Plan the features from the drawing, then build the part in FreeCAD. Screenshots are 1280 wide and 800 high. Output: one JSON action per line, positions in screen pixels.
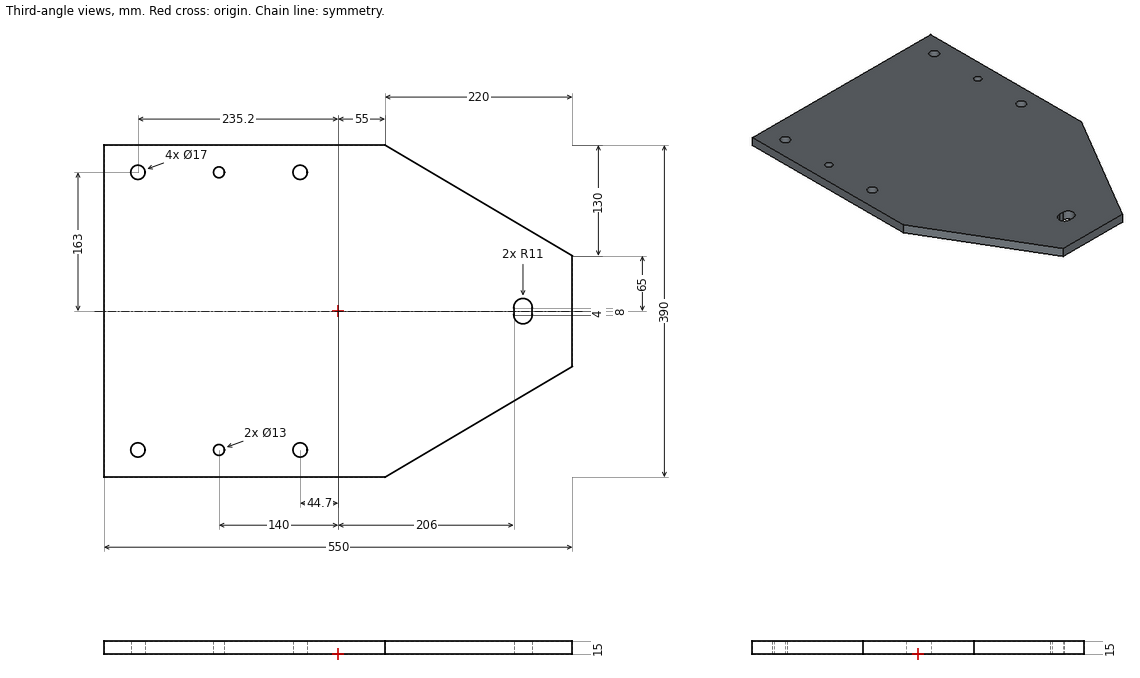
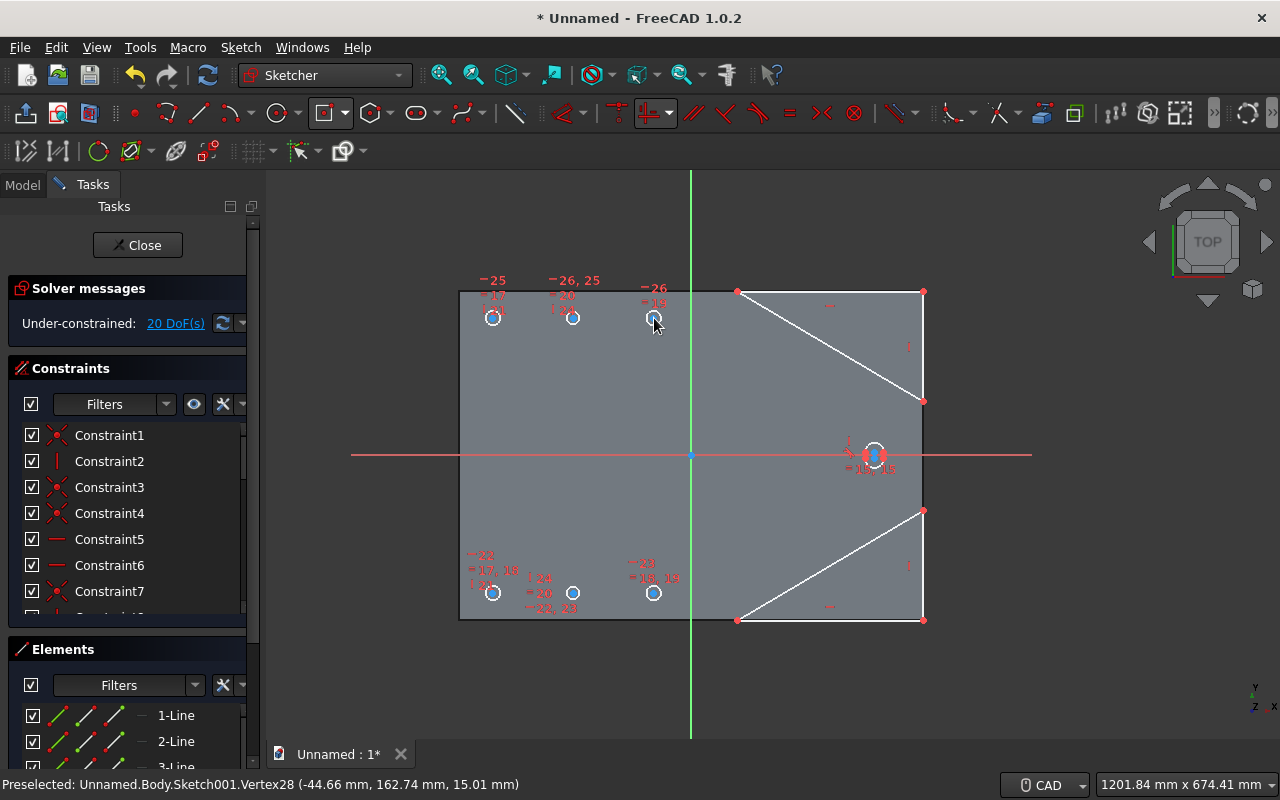
{"action": "left_click", "coordinate": [654, 593]}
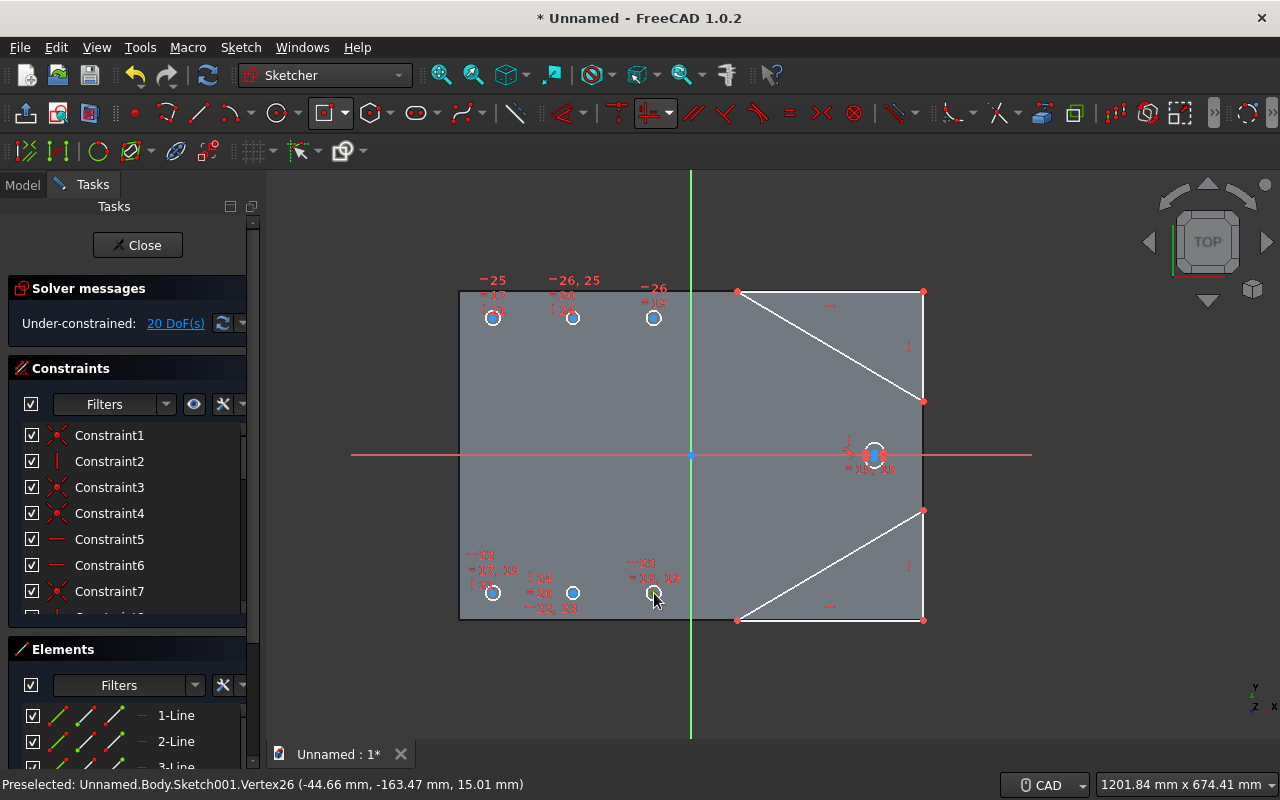
{"action": "left_click", "coordinate": [654, 318]}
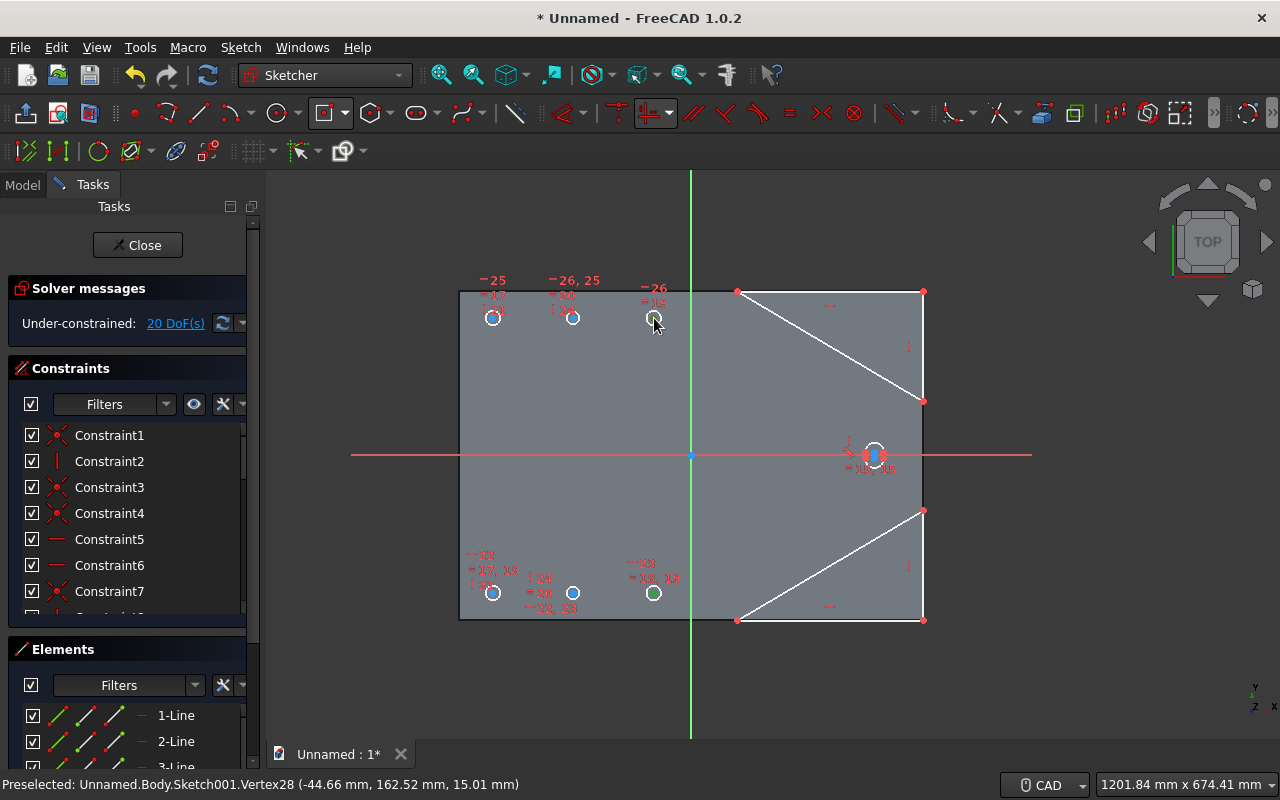
{"action": "left_click", "coordinate": [353, 455]}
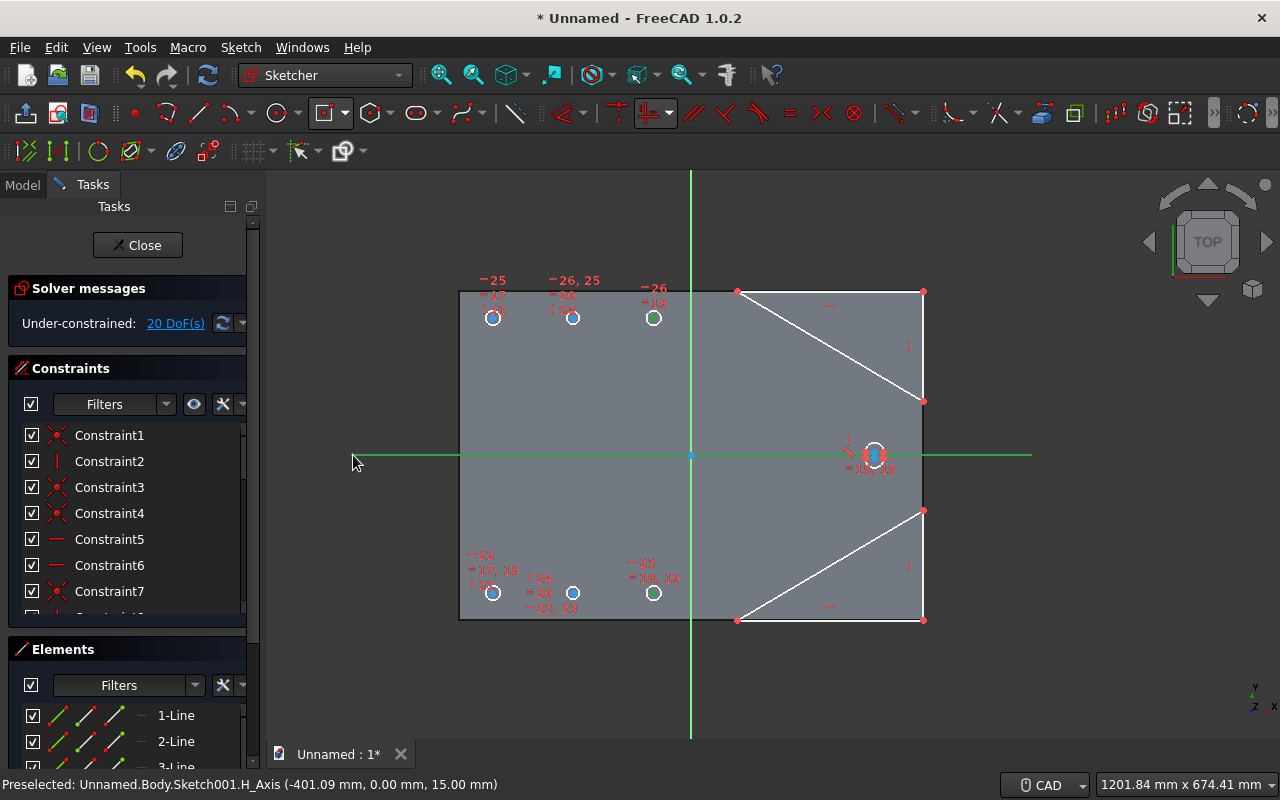
{"action": "left_click", "coordinate": [822, 114]}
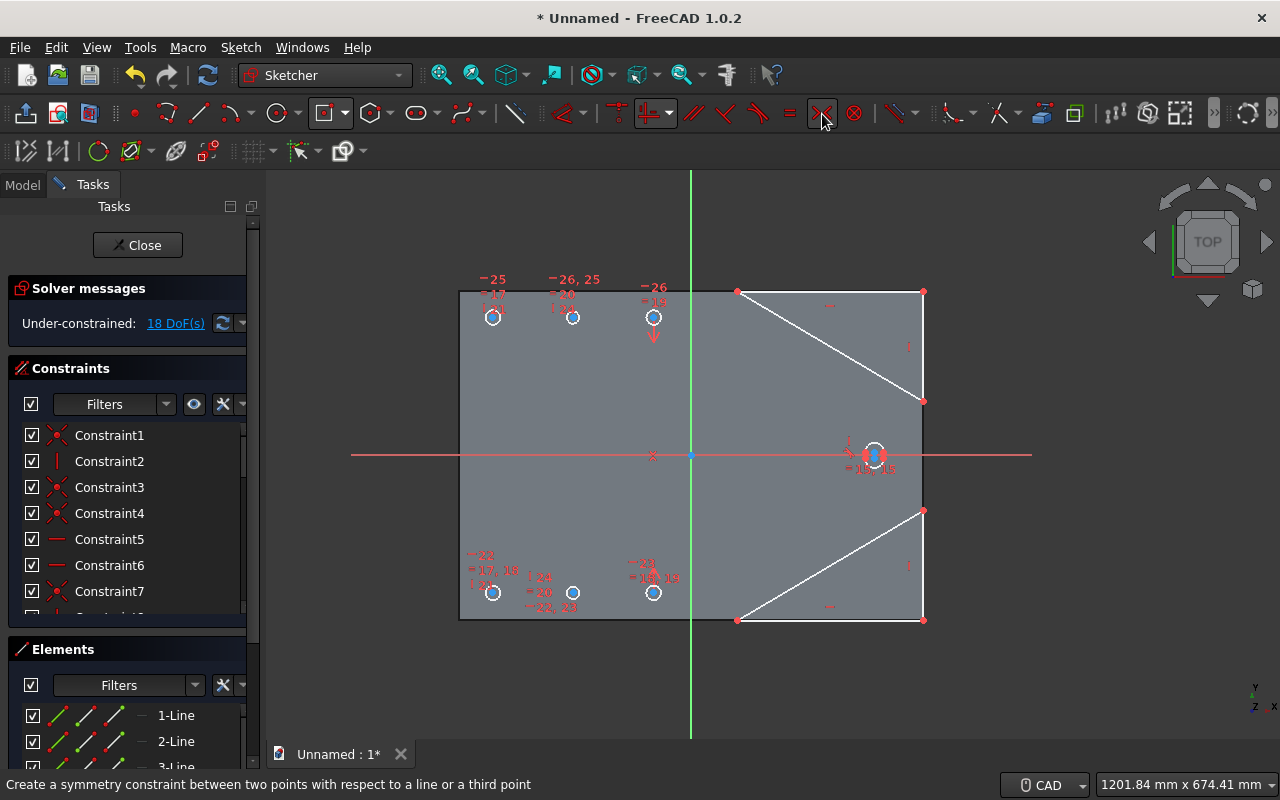
{"action": "left_click", "coordinate": [737, 292]}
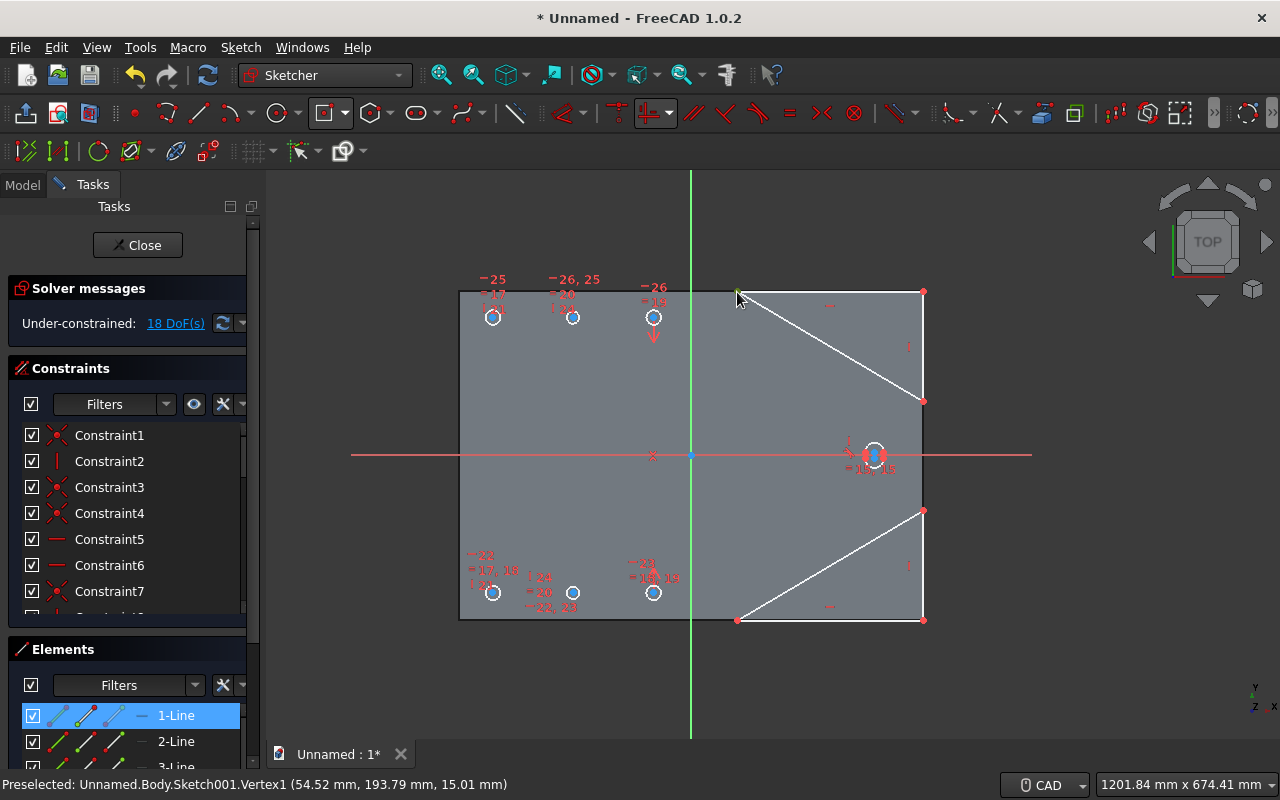
{"action": "left_click", "coordinate": [737, 621]}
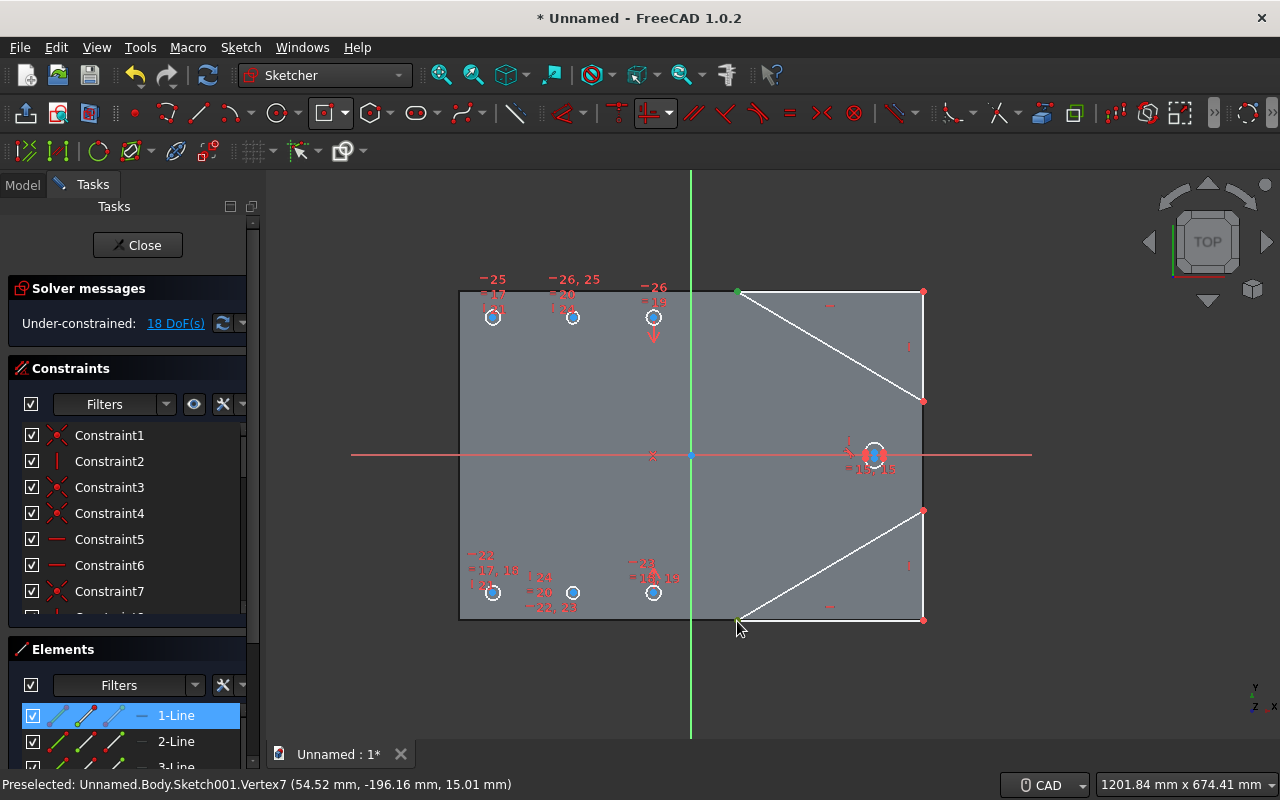
{"action": "left_click", "coordinate": [353, 455]}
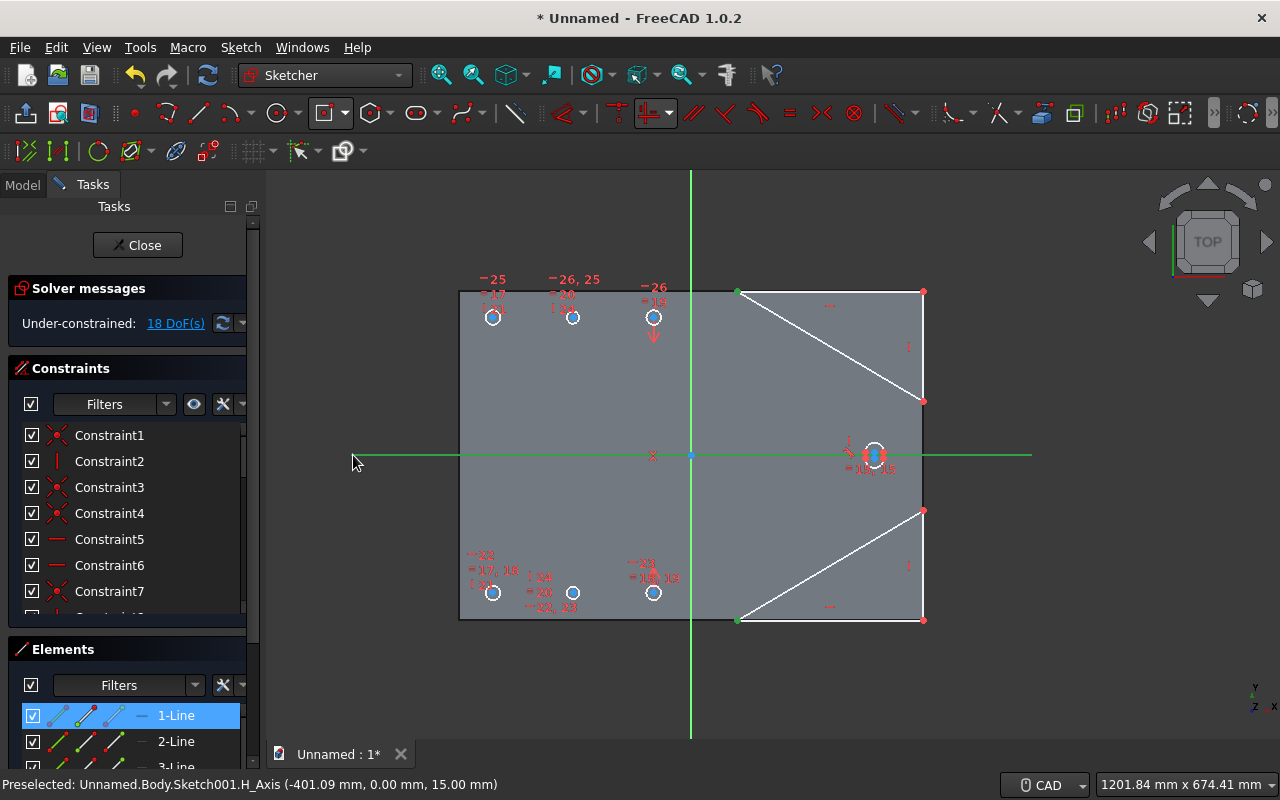
{"action": "left_click", "coordinate": [822, 114]}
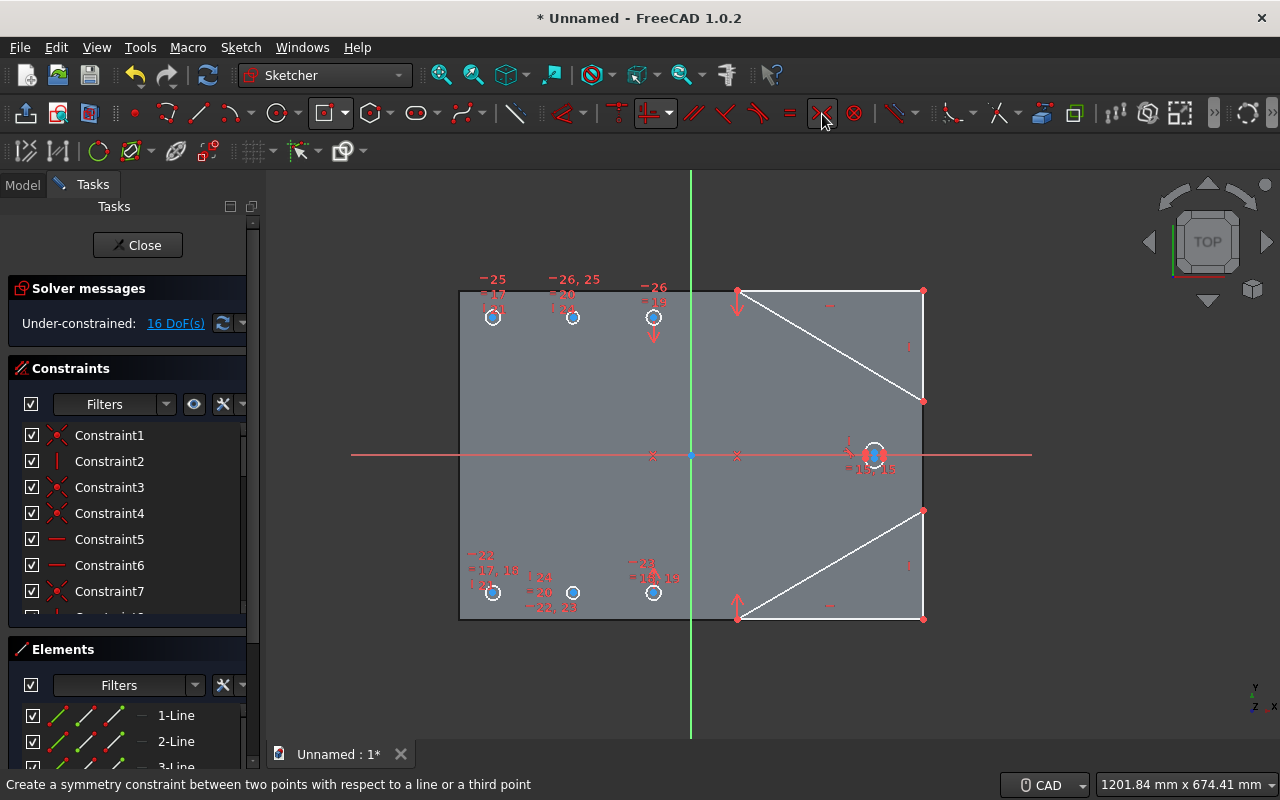
{"action": "left_click", "coordinate": [923, 402]}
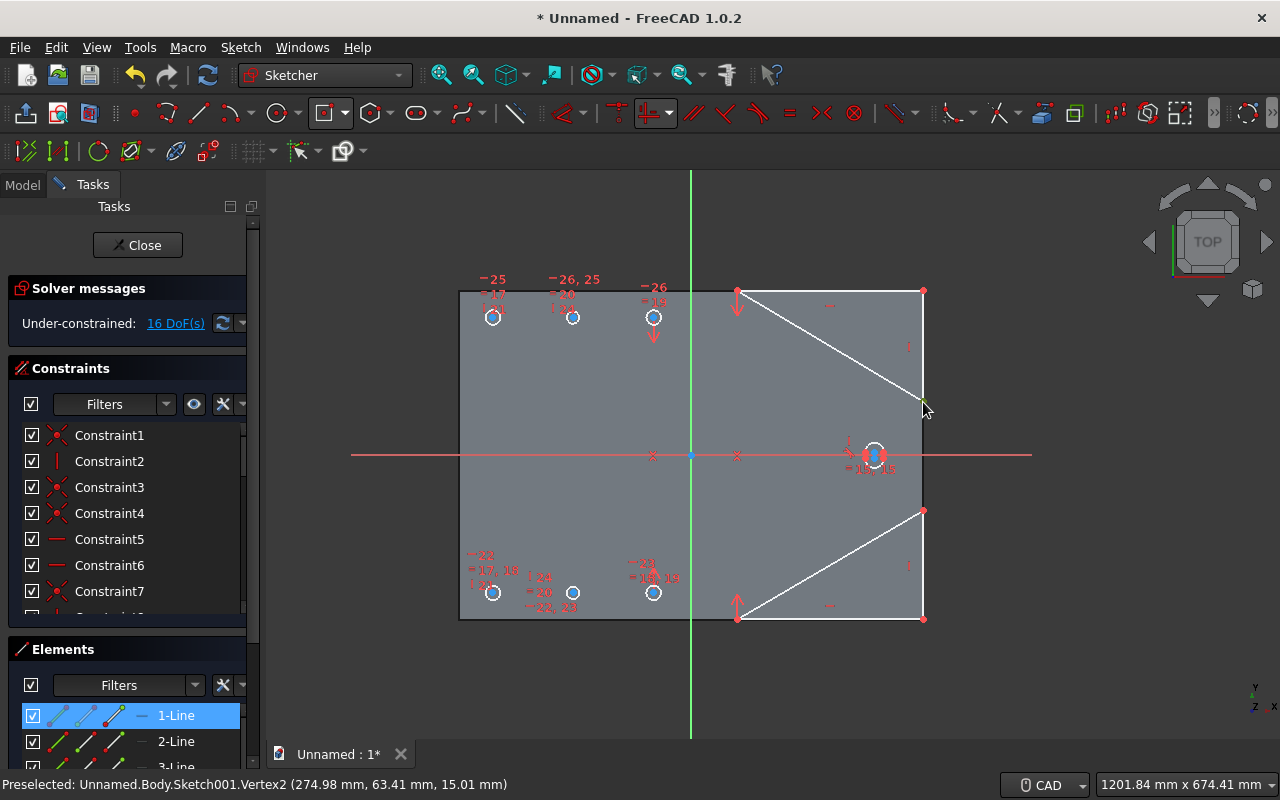
{"action": "left_click", "coordinate": [923, 511]}